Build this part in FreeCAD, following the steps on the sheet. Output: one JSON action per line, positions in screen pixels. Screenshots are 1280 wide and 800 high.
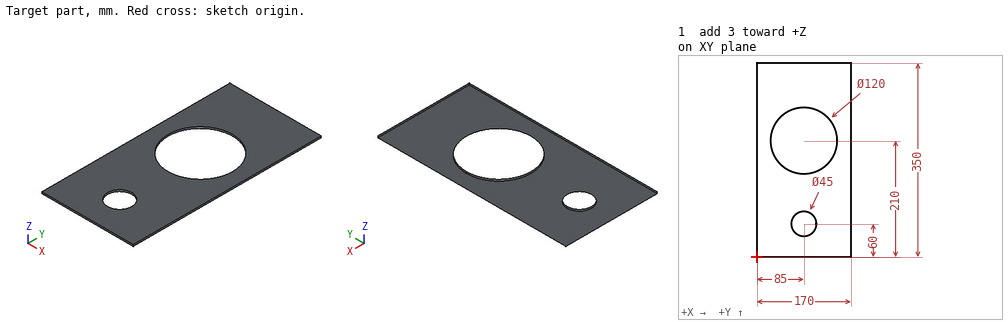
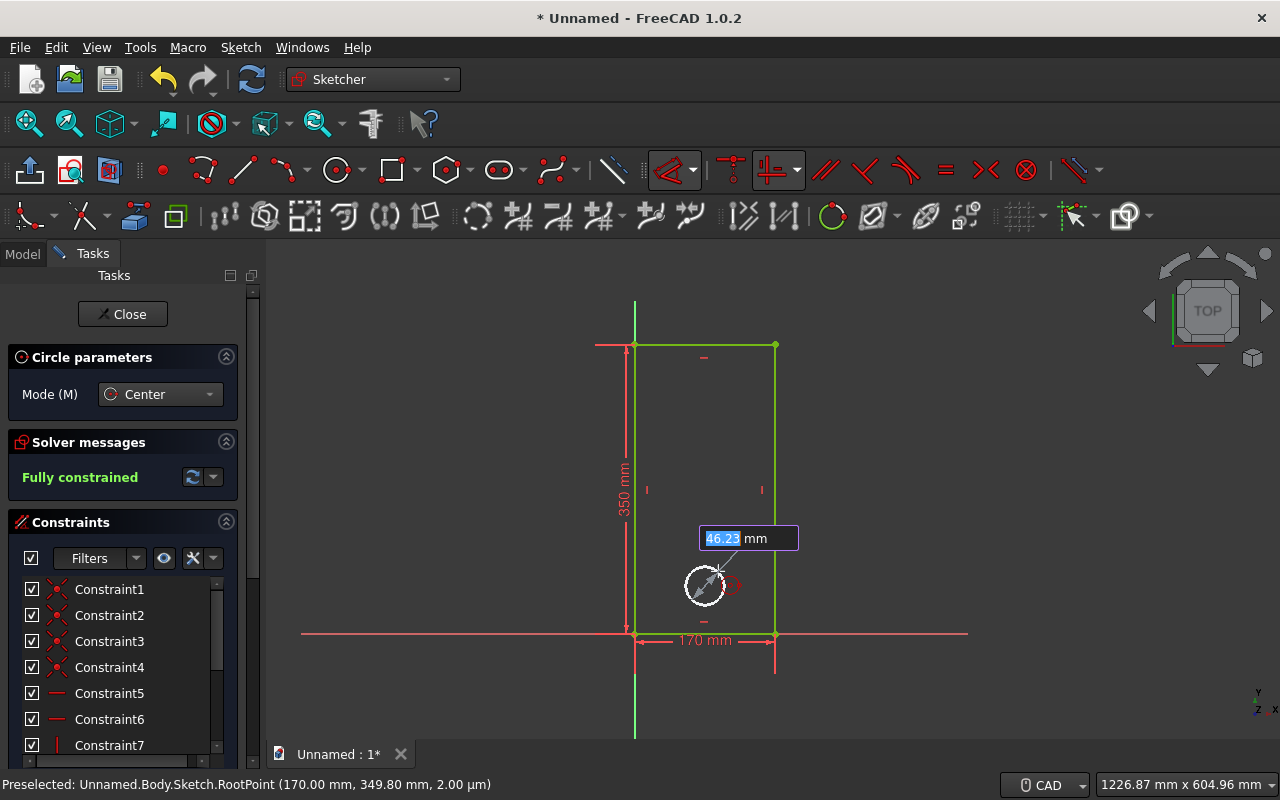
{"action": "type", "text": "45"}
{"action": "key", "text": "Return"}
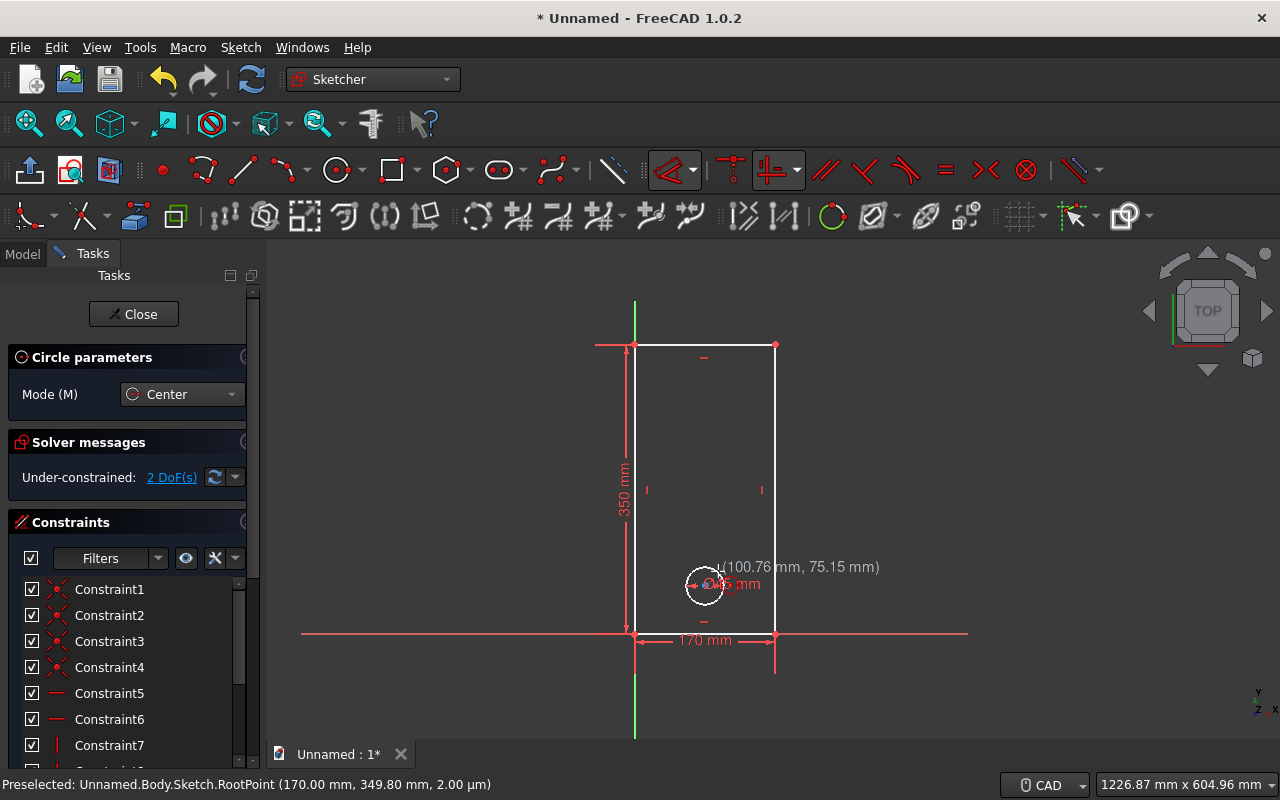
{"action": "left_click", "coordinate": [705, 461]}
{"action": "mouse_move", "coordinate": [740, 425]}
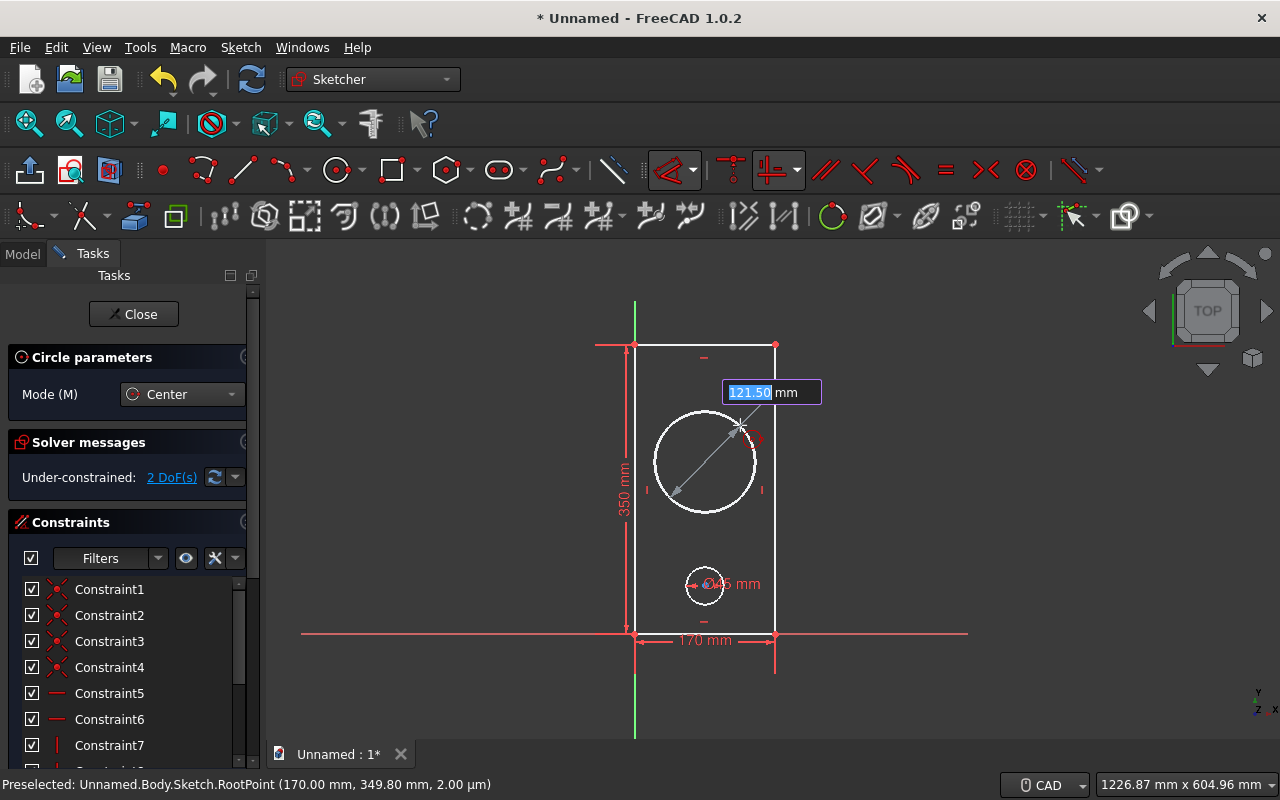
{"action": "type", "text": "120"}
{"action": "key", "text": "Return"}
{"action": "key", "text": "Escape"}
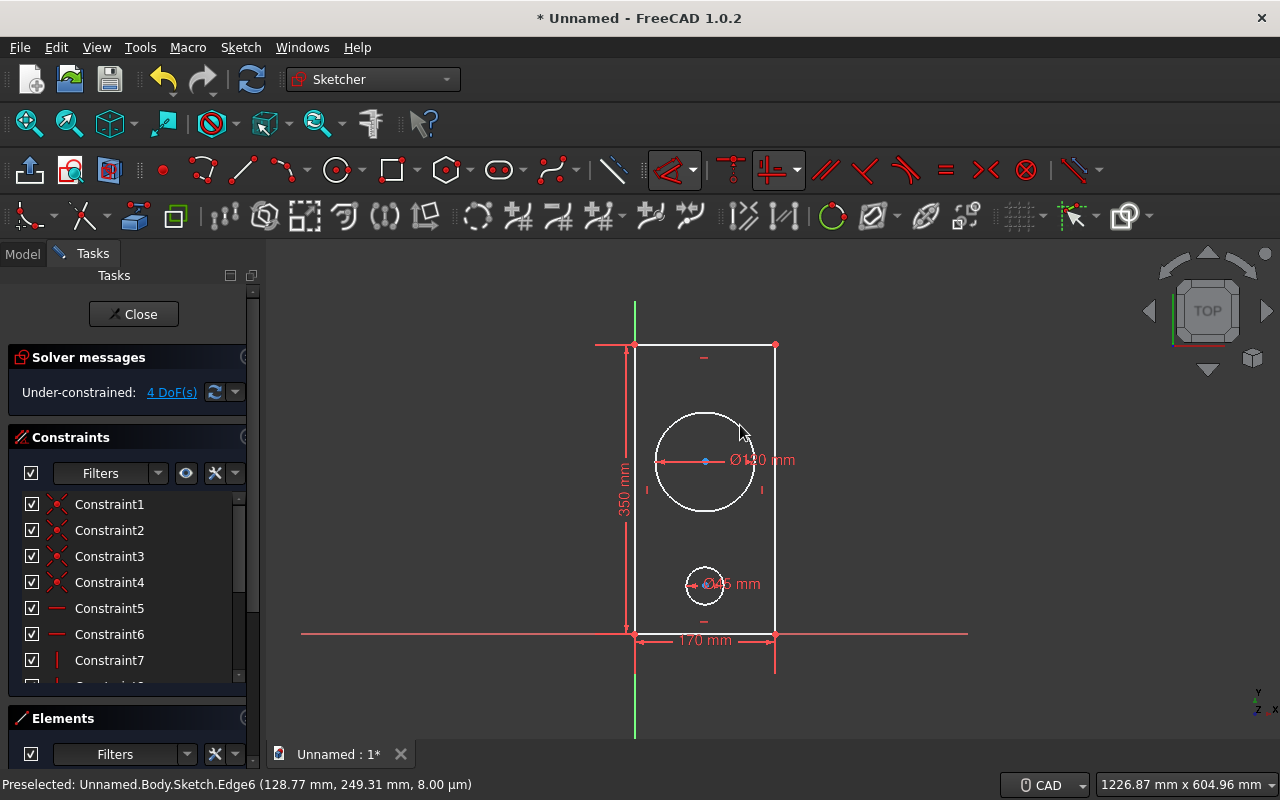
{"action": "left_click", "coordinate": [705, 586]}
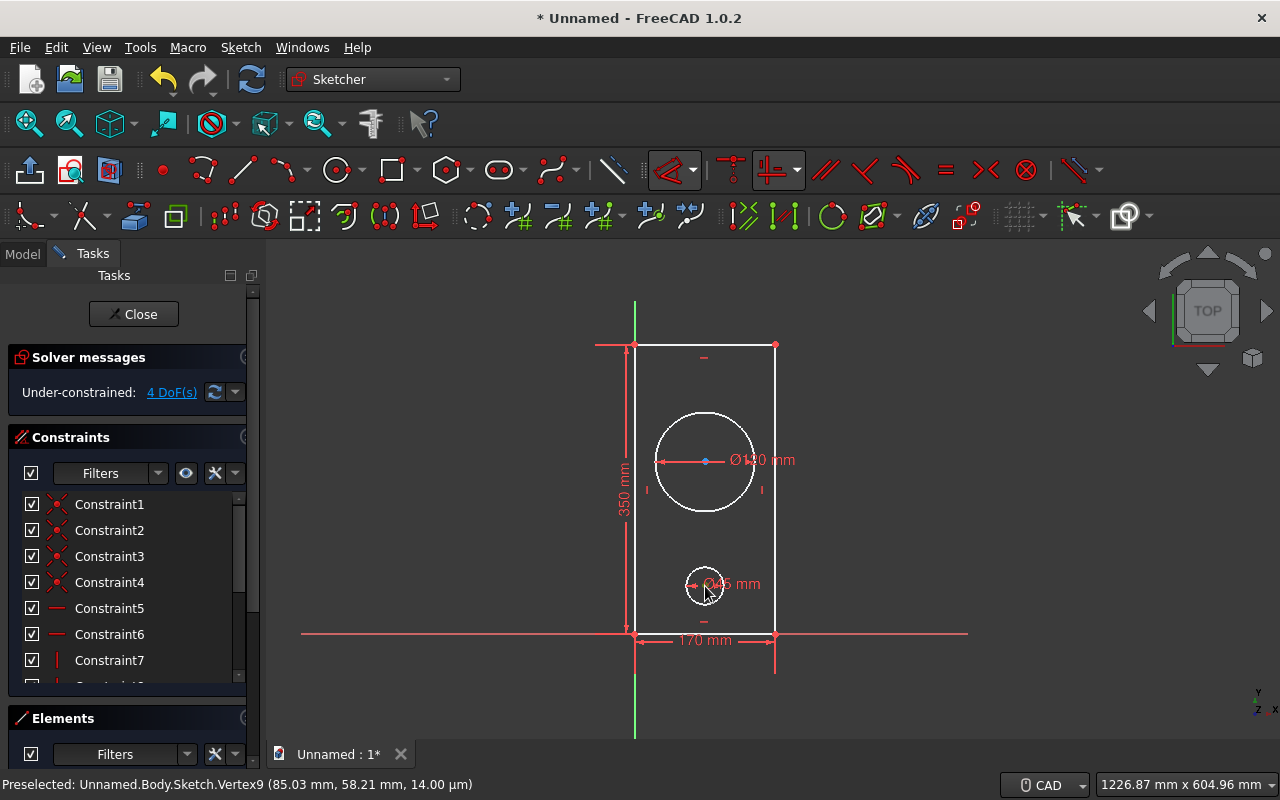
{"action": "left_click", "coordinate": [705, 462]}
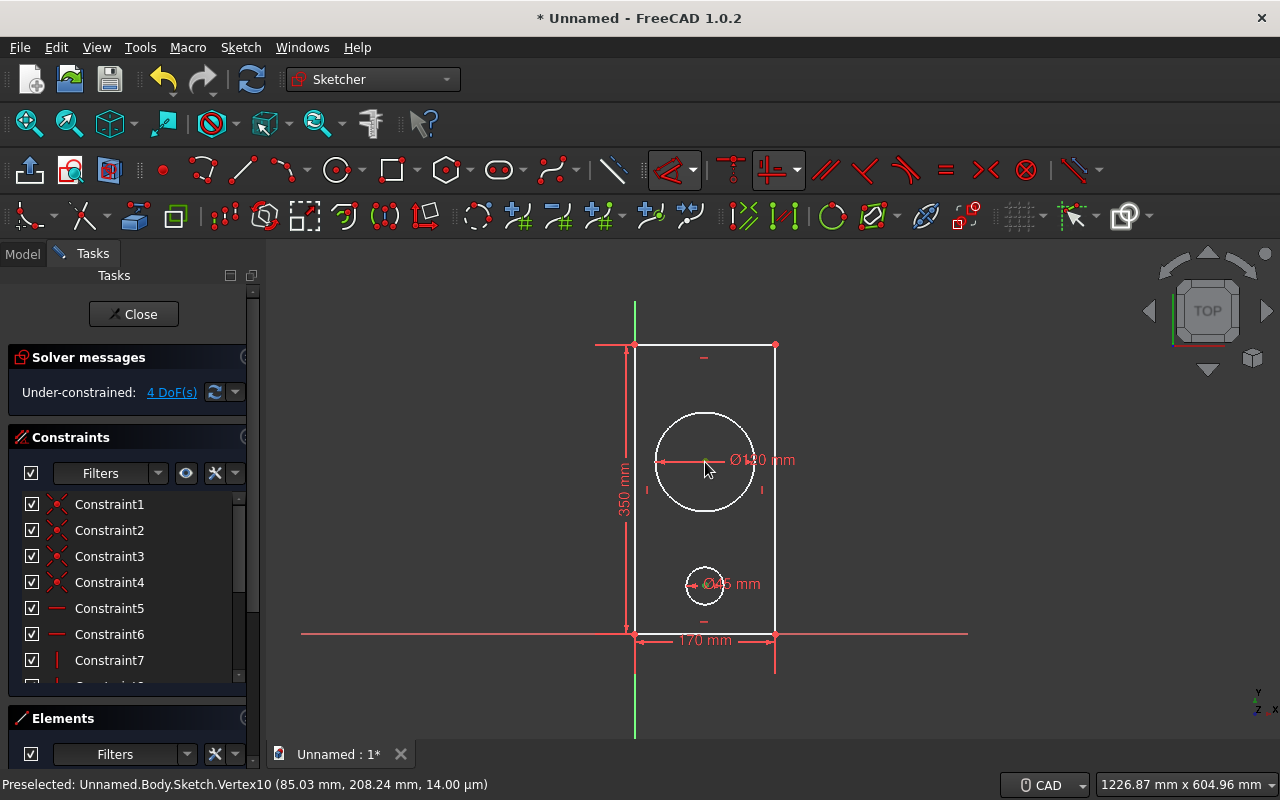
{"action": "key", "text": "v"}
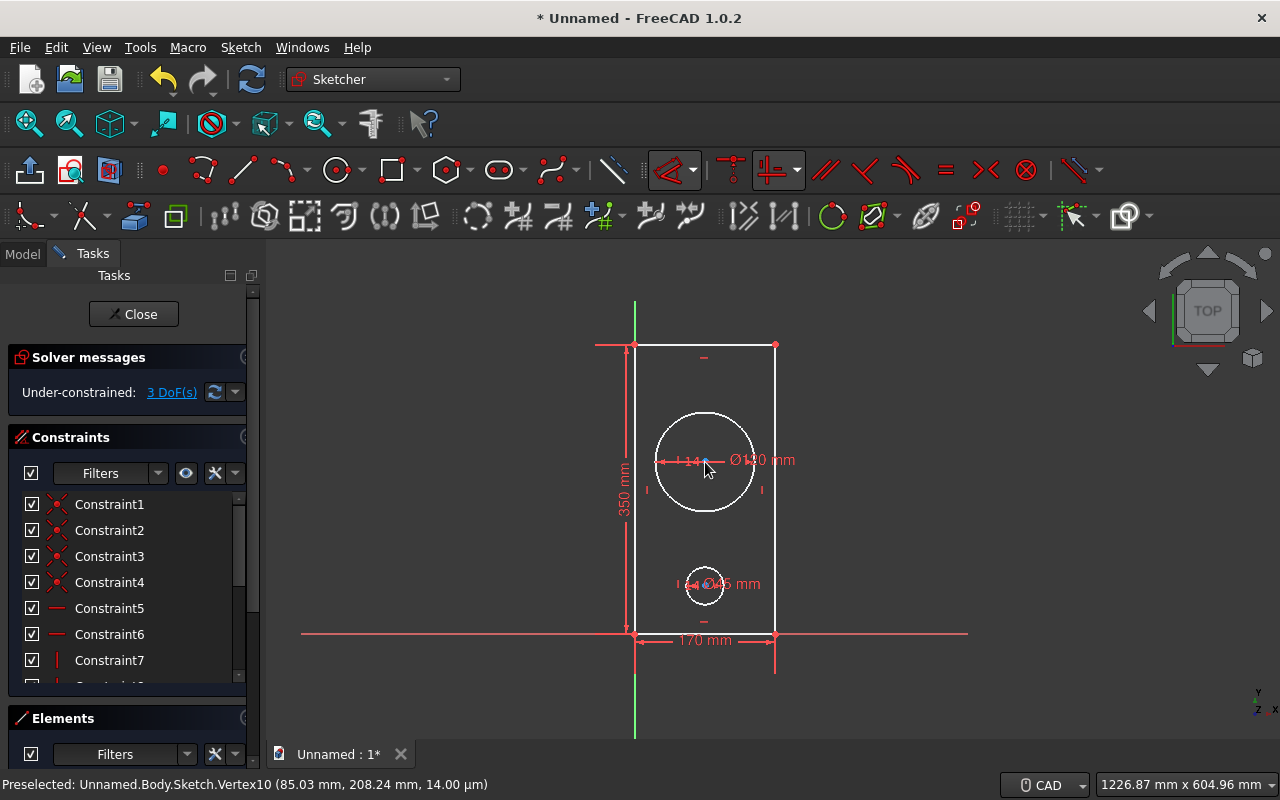
{"action": "left_click", "coordinate": [668, 170]}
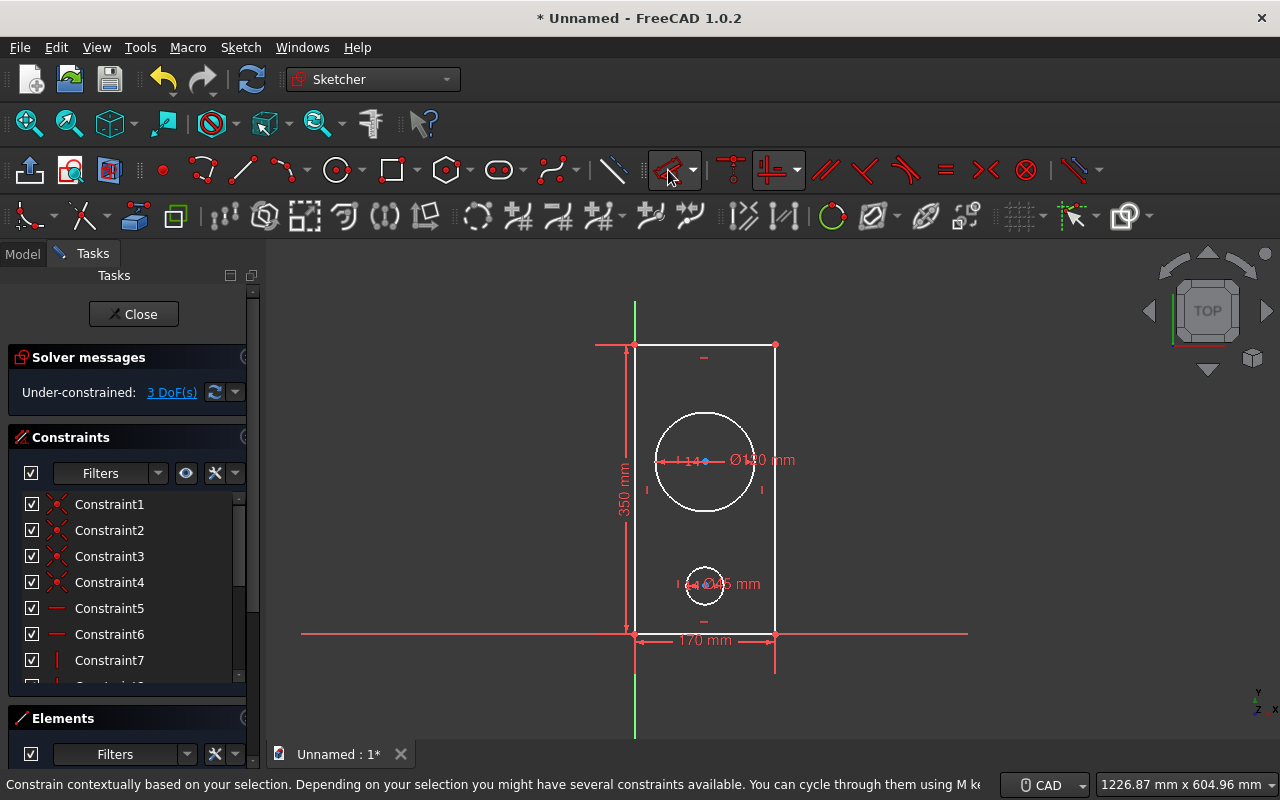
{"action": "left_click", "coordinate": [705, 586]}
{"action": "left_click", "coordinate": [670, 668]}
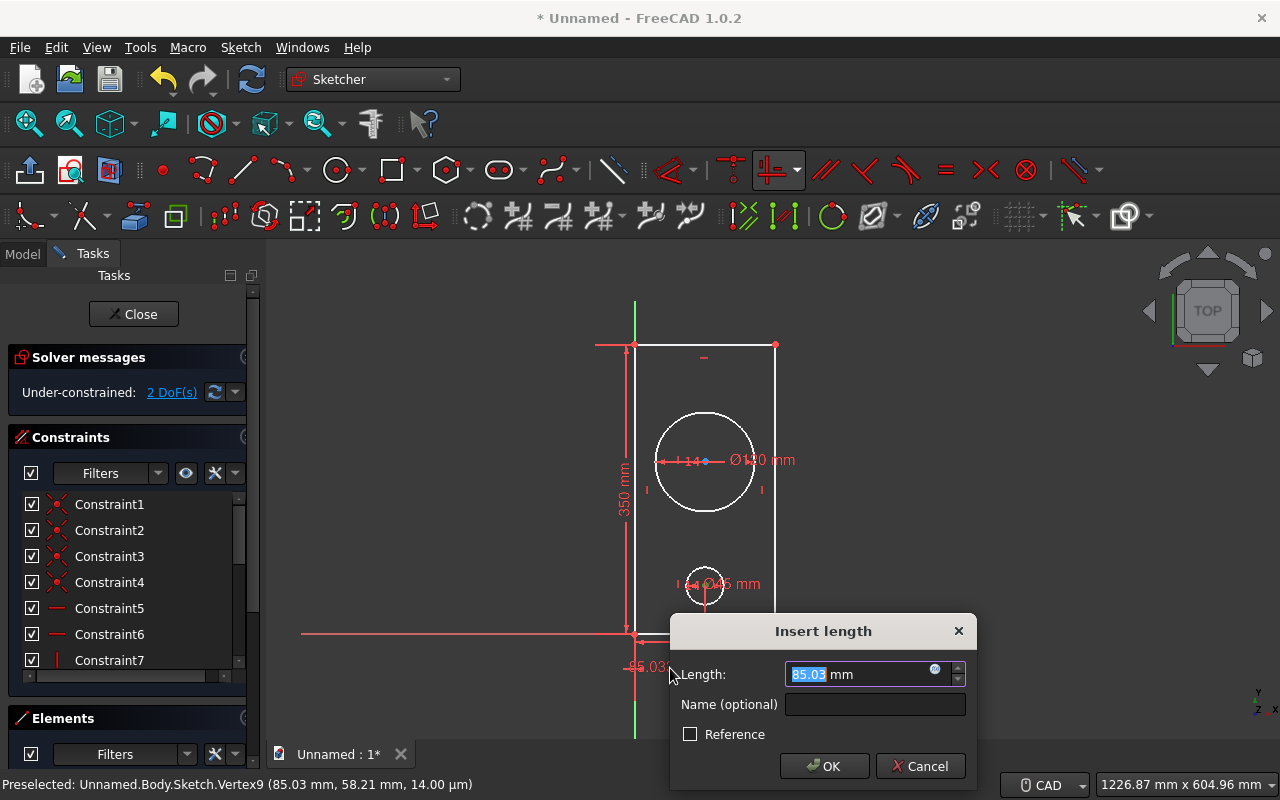
{"action": "type", "text": "85"}
{"action": "key", "text": "Return"}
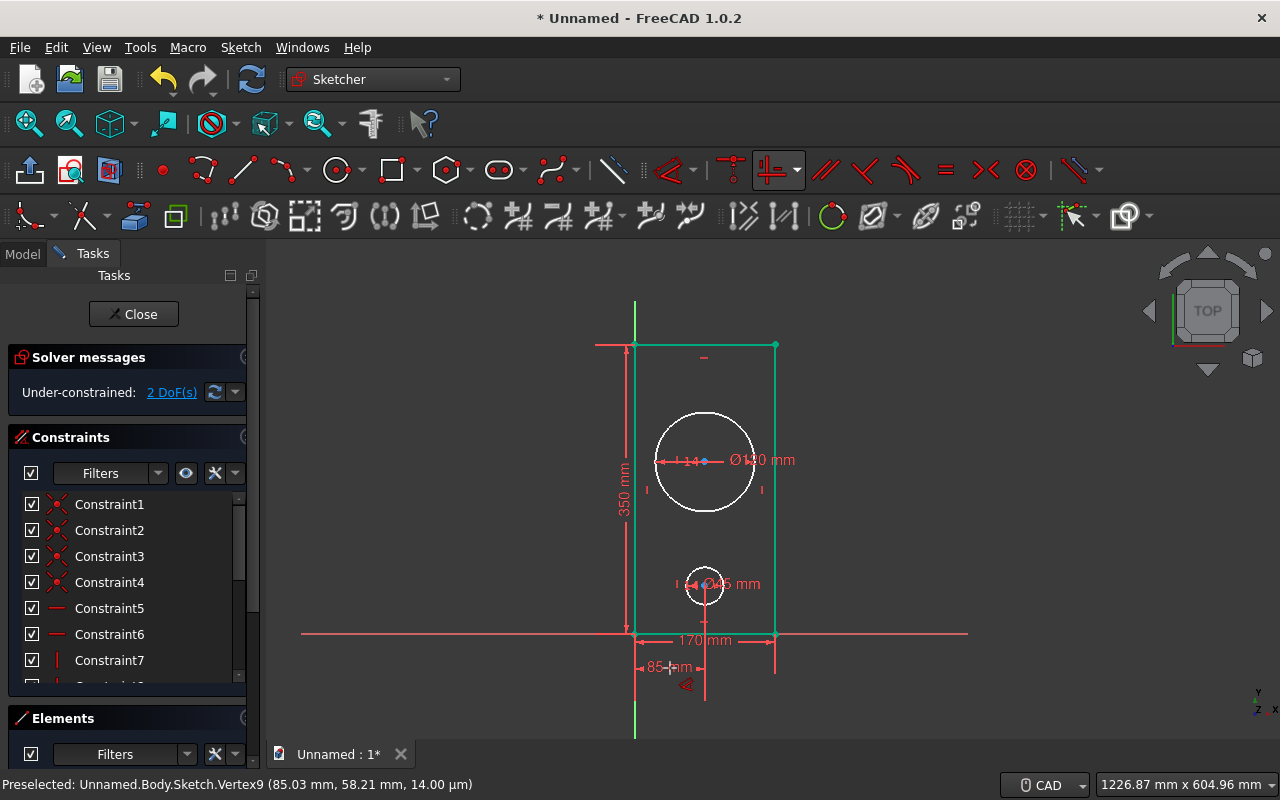
{"action": "left_click", "coordinate": [705, 586]}
{"action": "left_click", "coordinate": [601, 610]}